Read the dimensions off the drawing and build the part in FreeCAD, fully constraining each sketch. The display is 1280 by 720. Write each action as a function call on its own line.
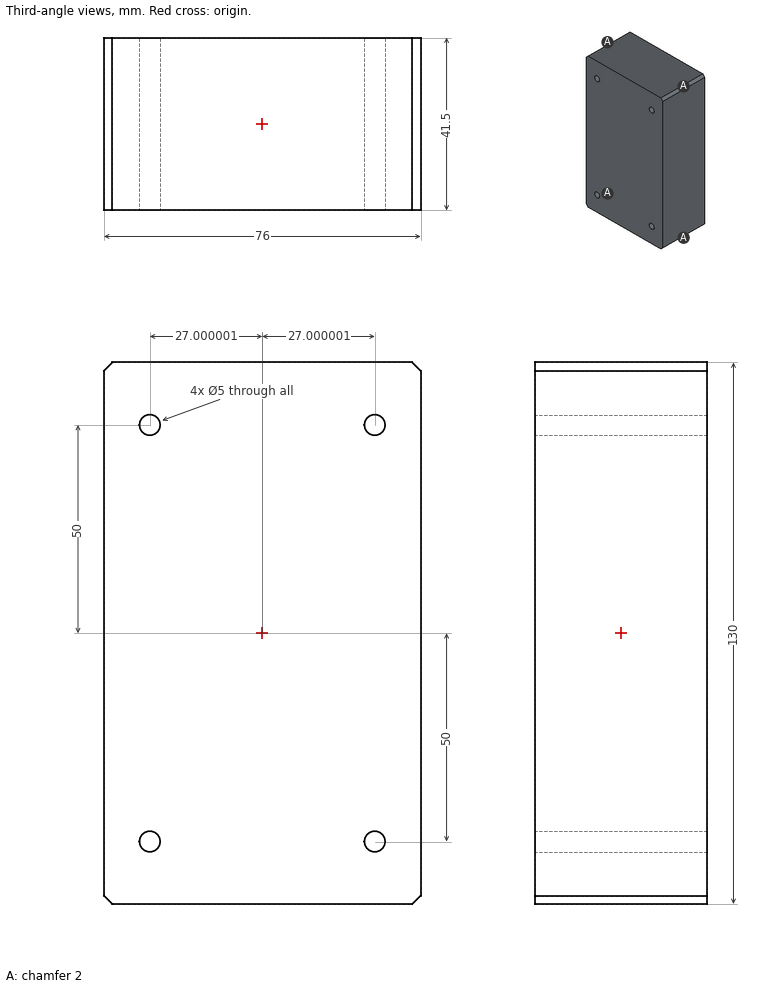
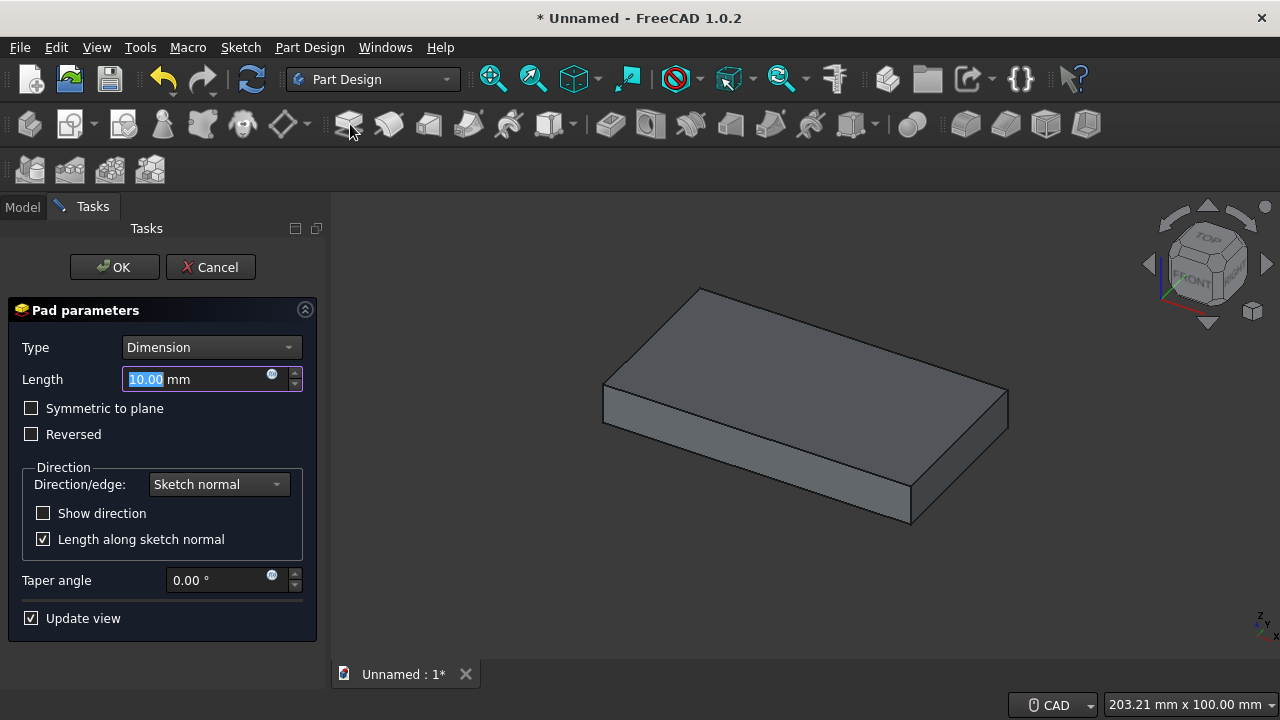
text(130)
key(Tab)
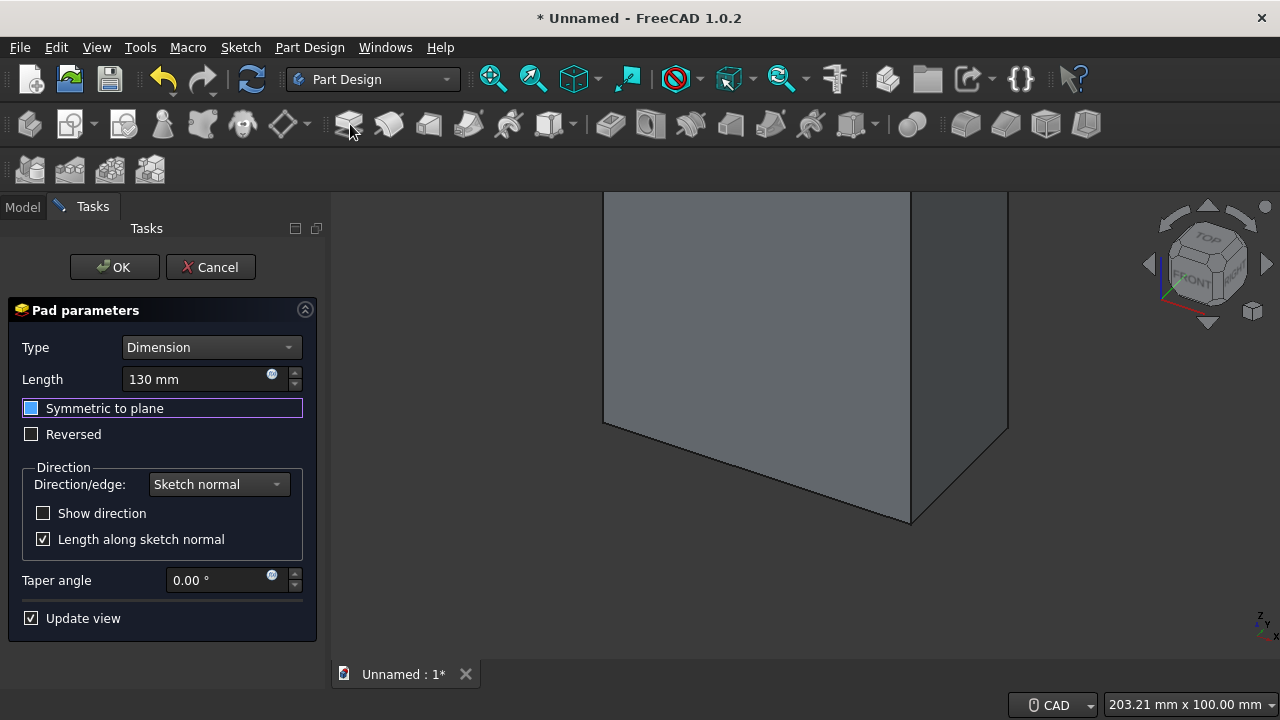
click(30, 408)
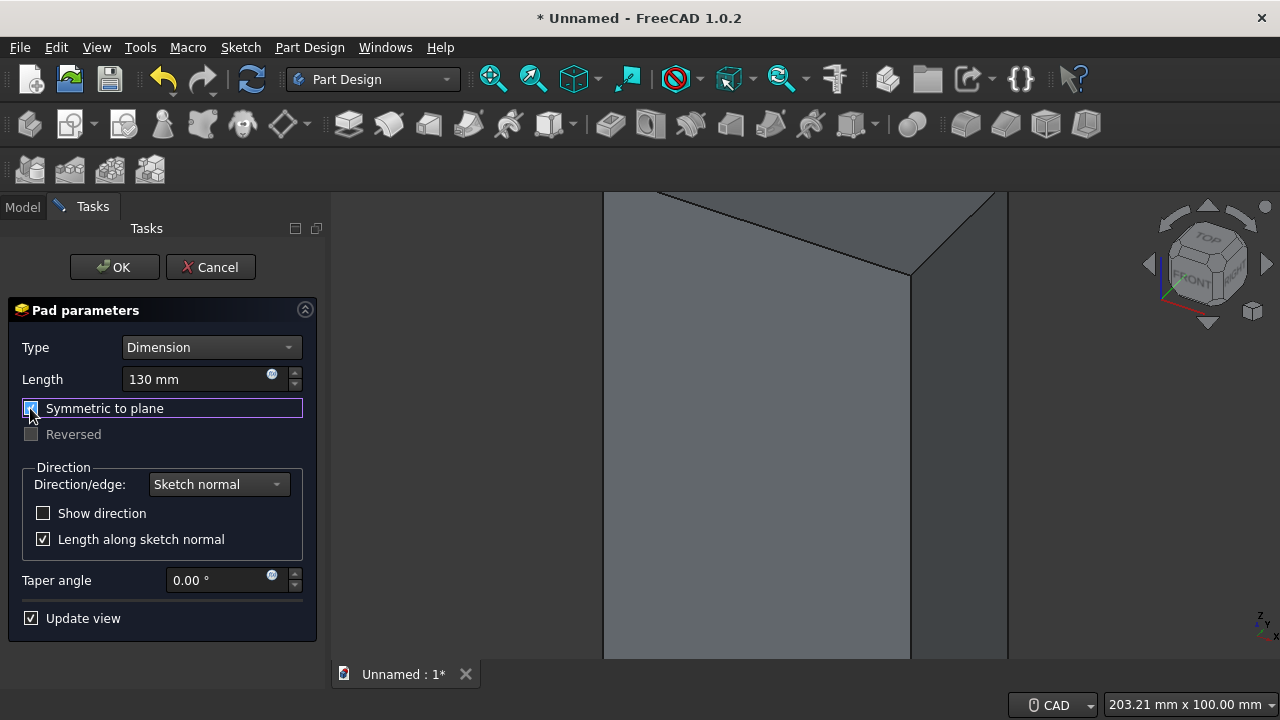
click(115, 267)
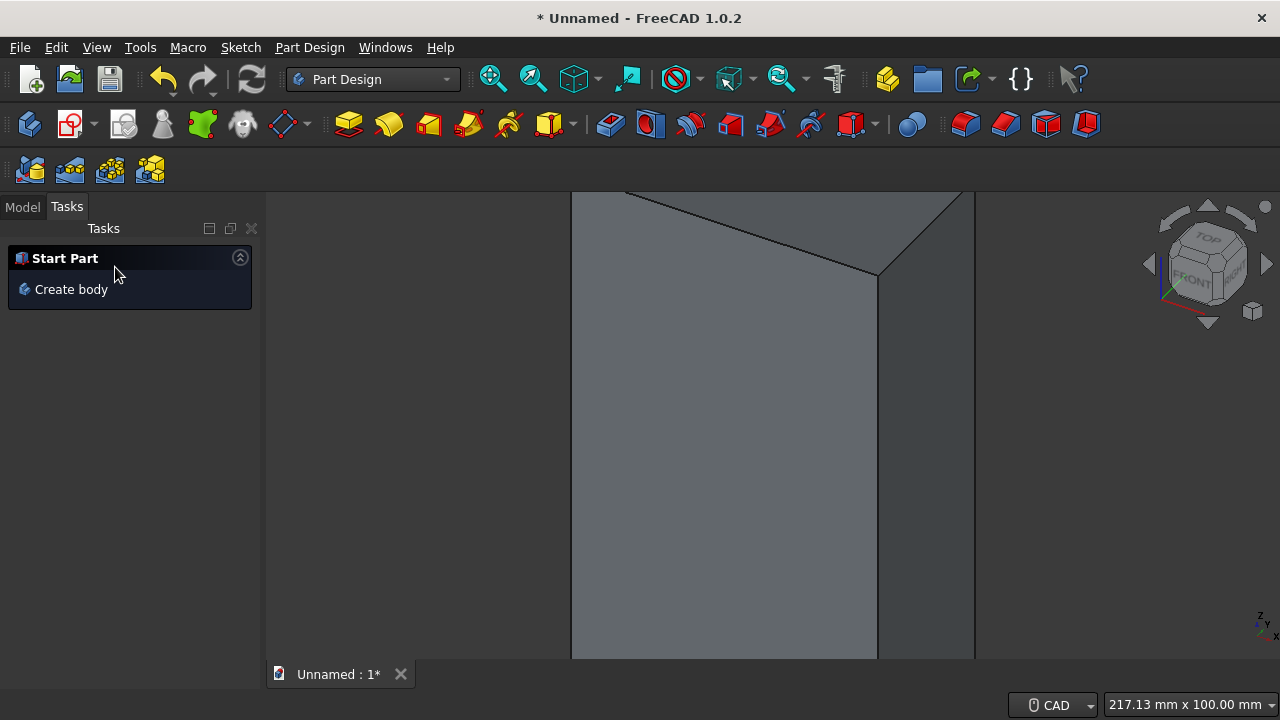
click(494, 80)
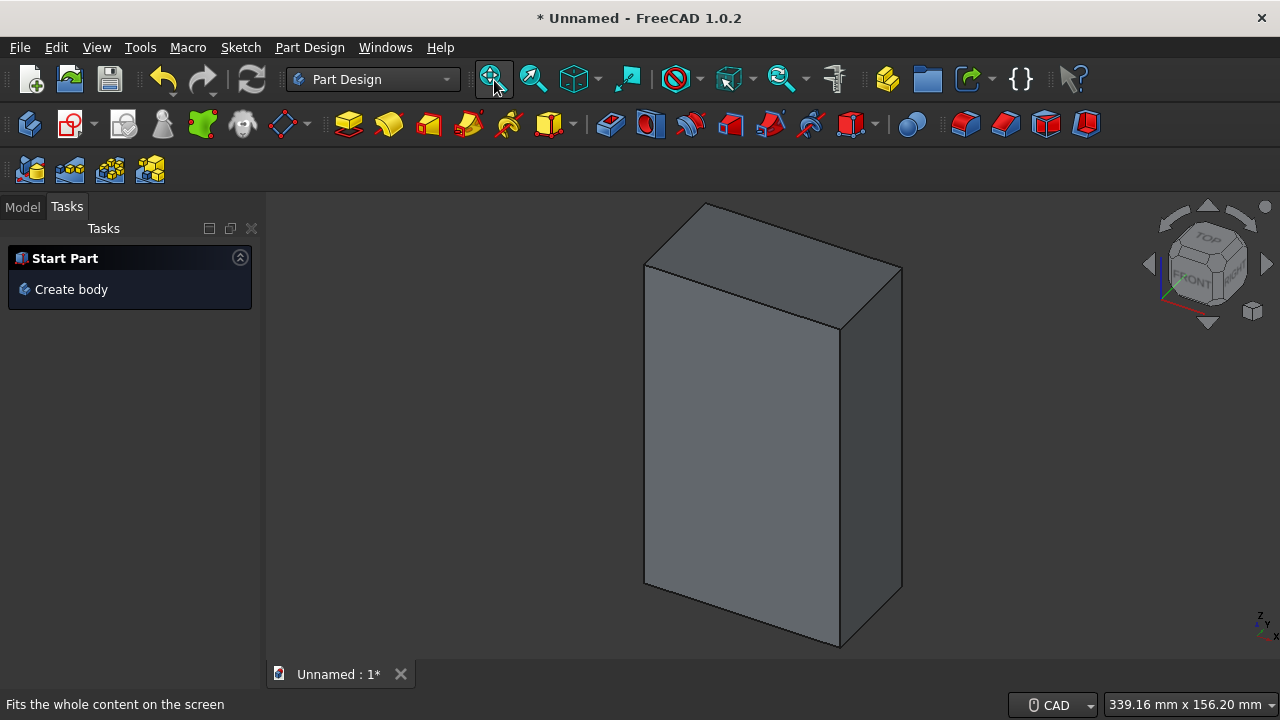
key(4)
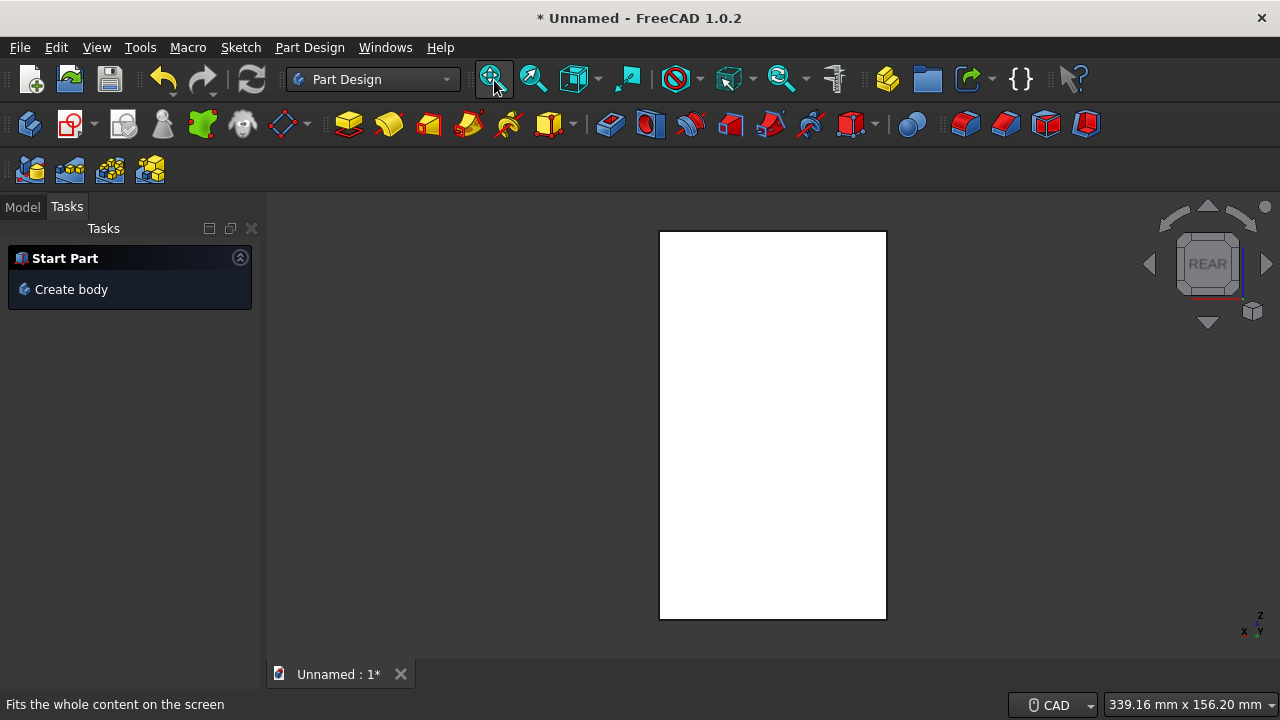
click(773, 369)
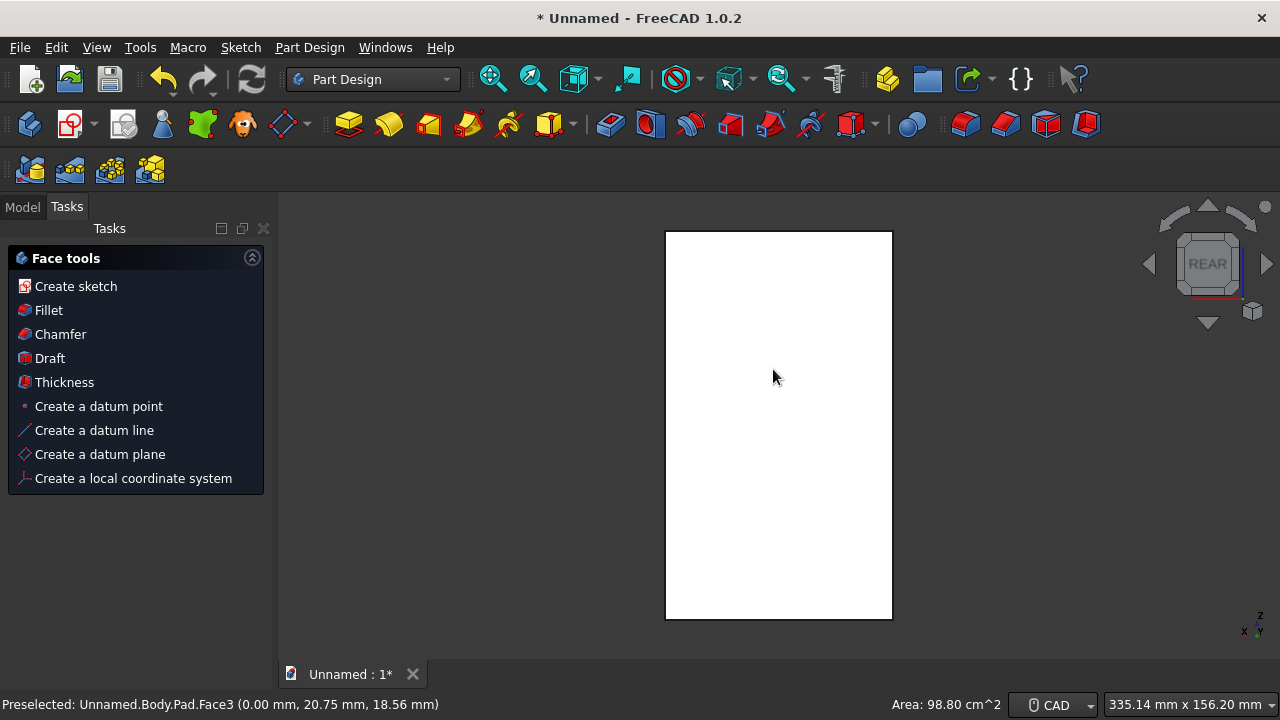
click(70, 124)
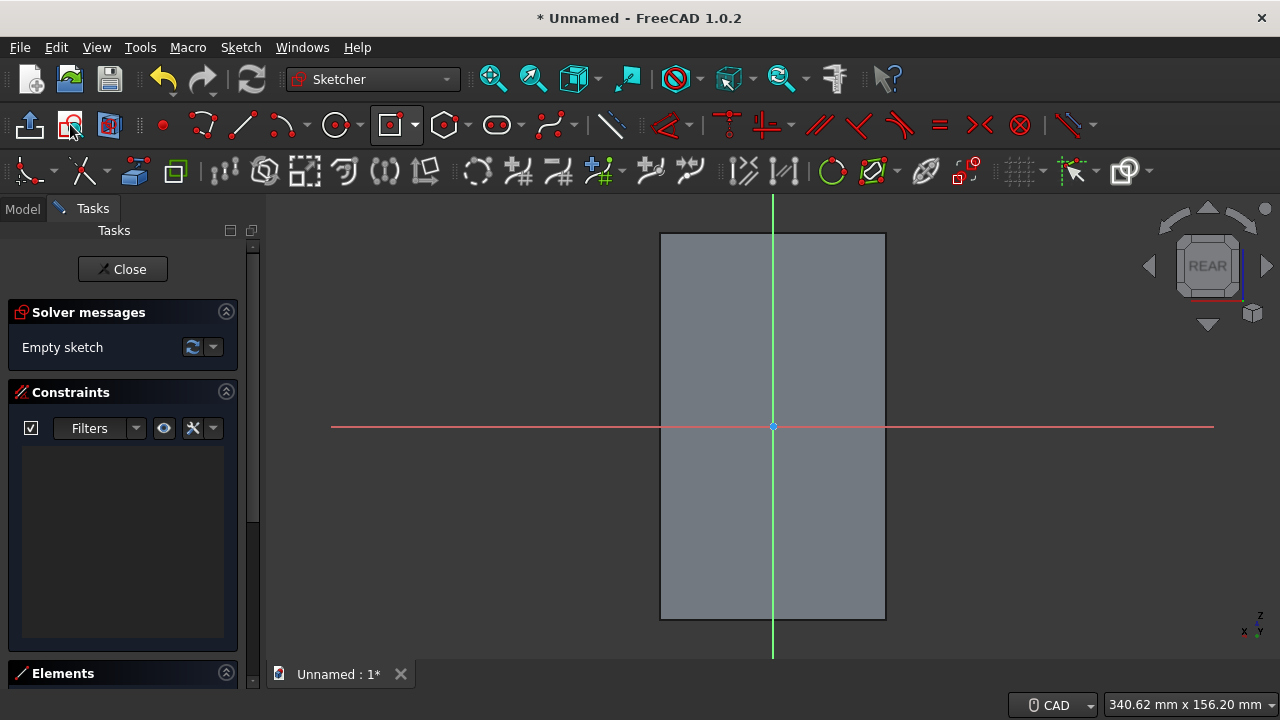
click(336, 126)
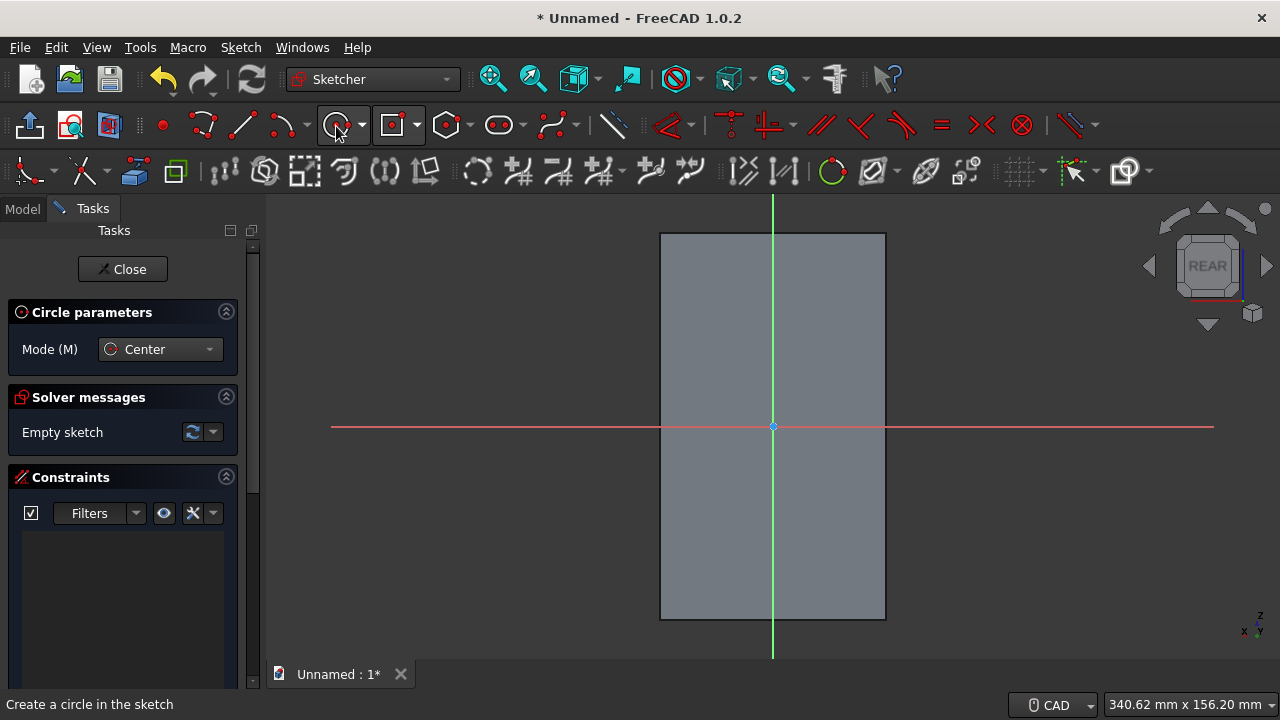
scroll(853, 278, up, 6)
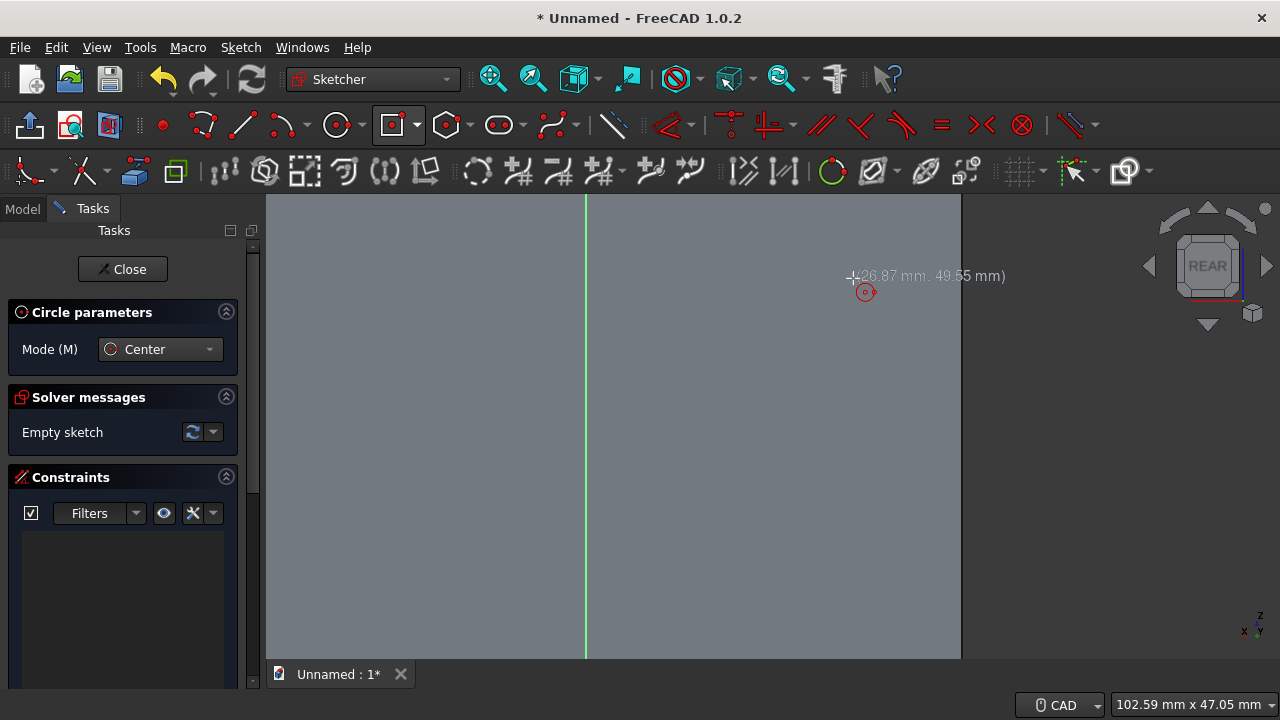
click(853, 276)
move(870, 259)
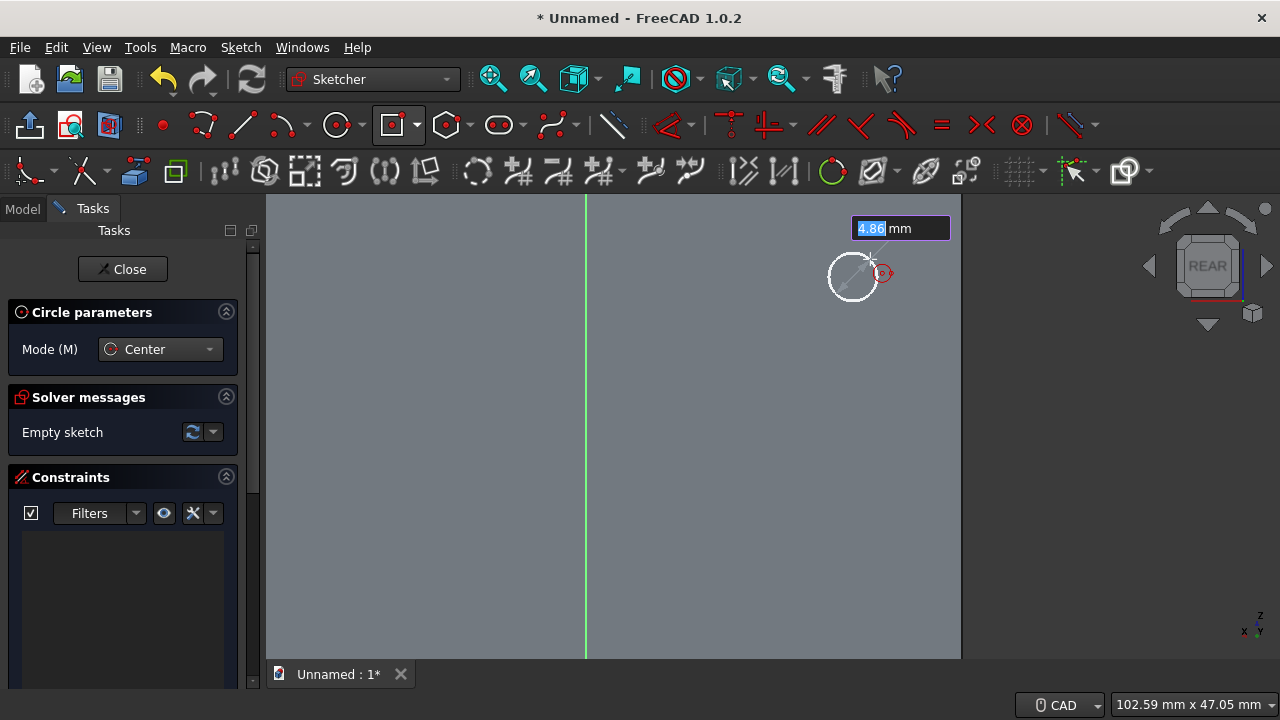
text(5)
key(Return)